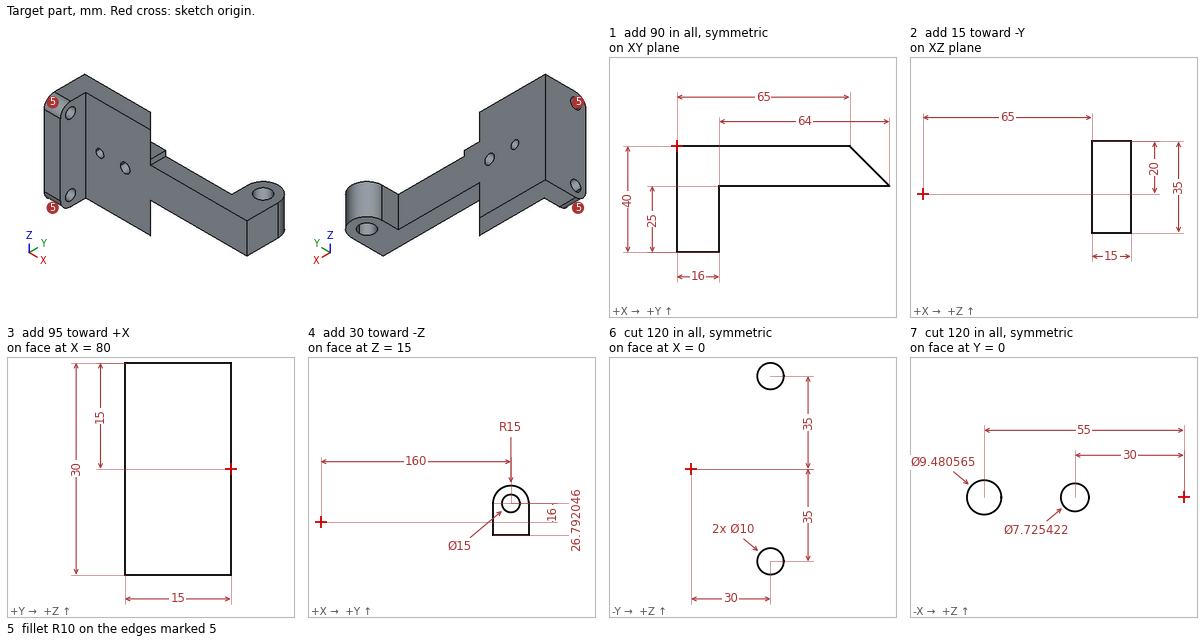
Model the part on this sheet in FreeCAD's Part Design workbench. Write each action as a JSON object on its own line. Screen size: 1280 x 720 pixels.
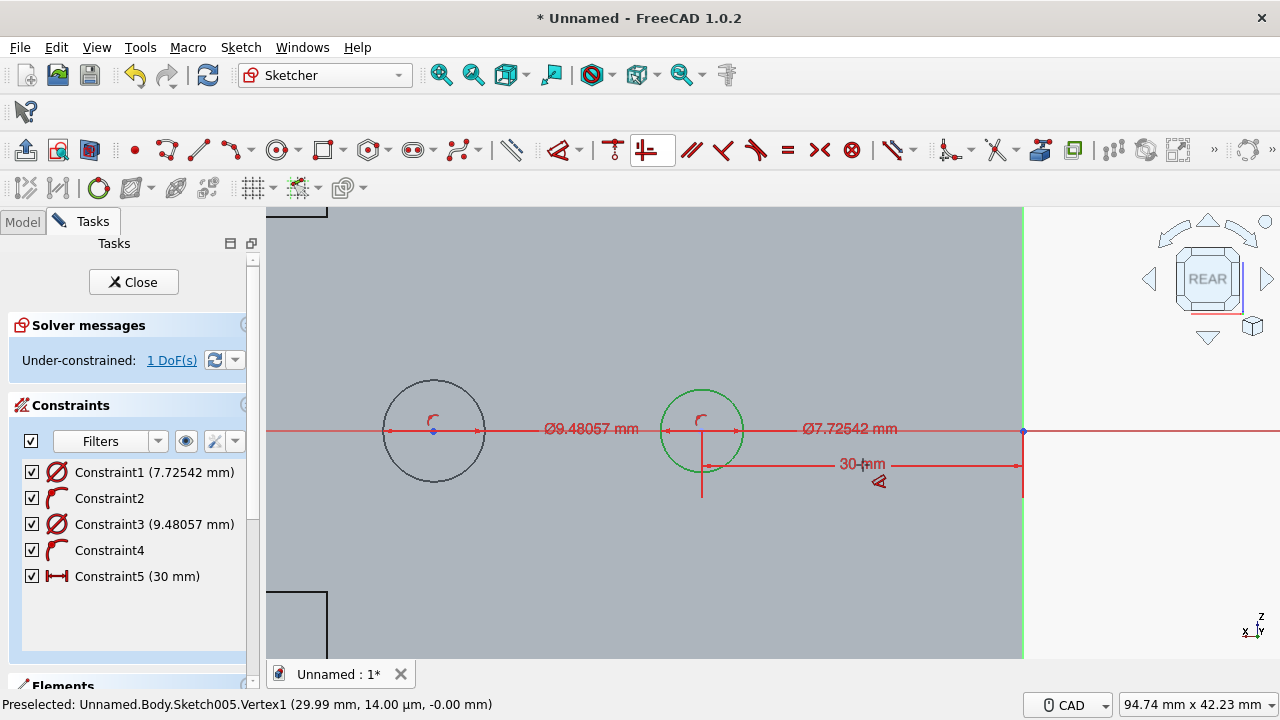
{"action": "left_click", "coordinate": [434, 431]}
{"action": "left_click", "coordinate": [593, 465]}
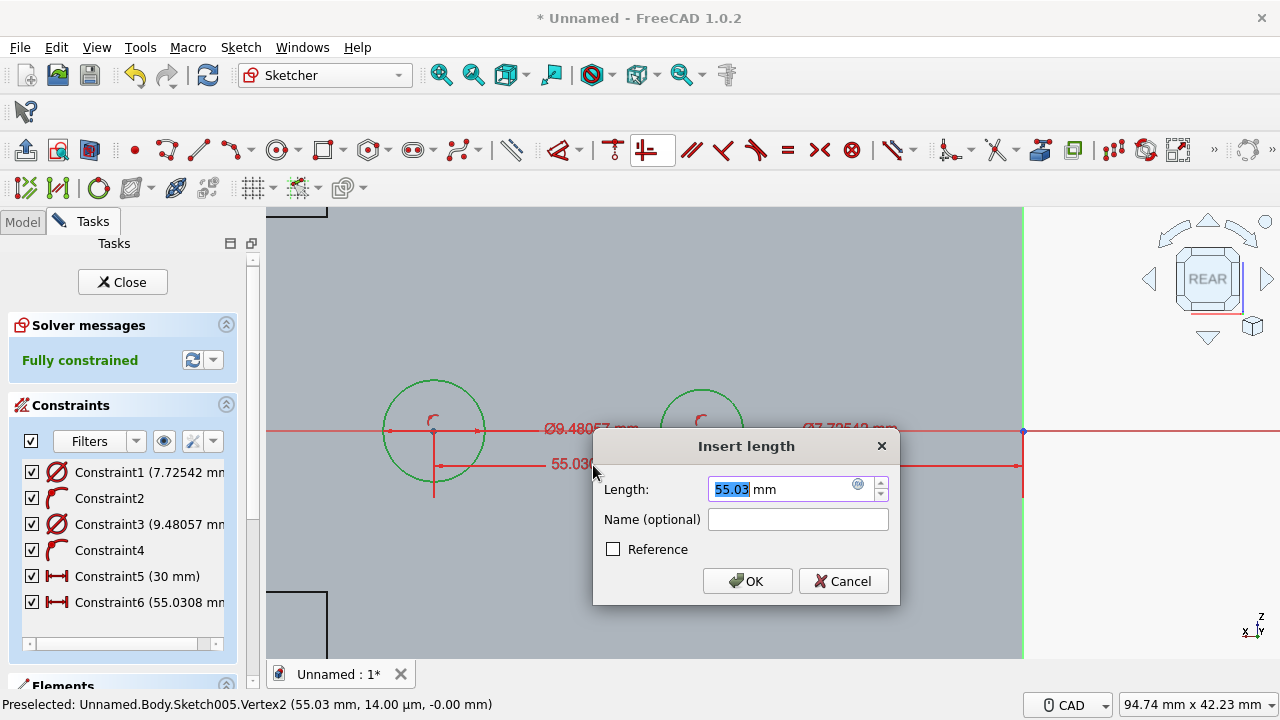
{"action": "type", "text": "55"}
{"action": "key", "text": "Return"}
{"action": "key", "text": "Escape"}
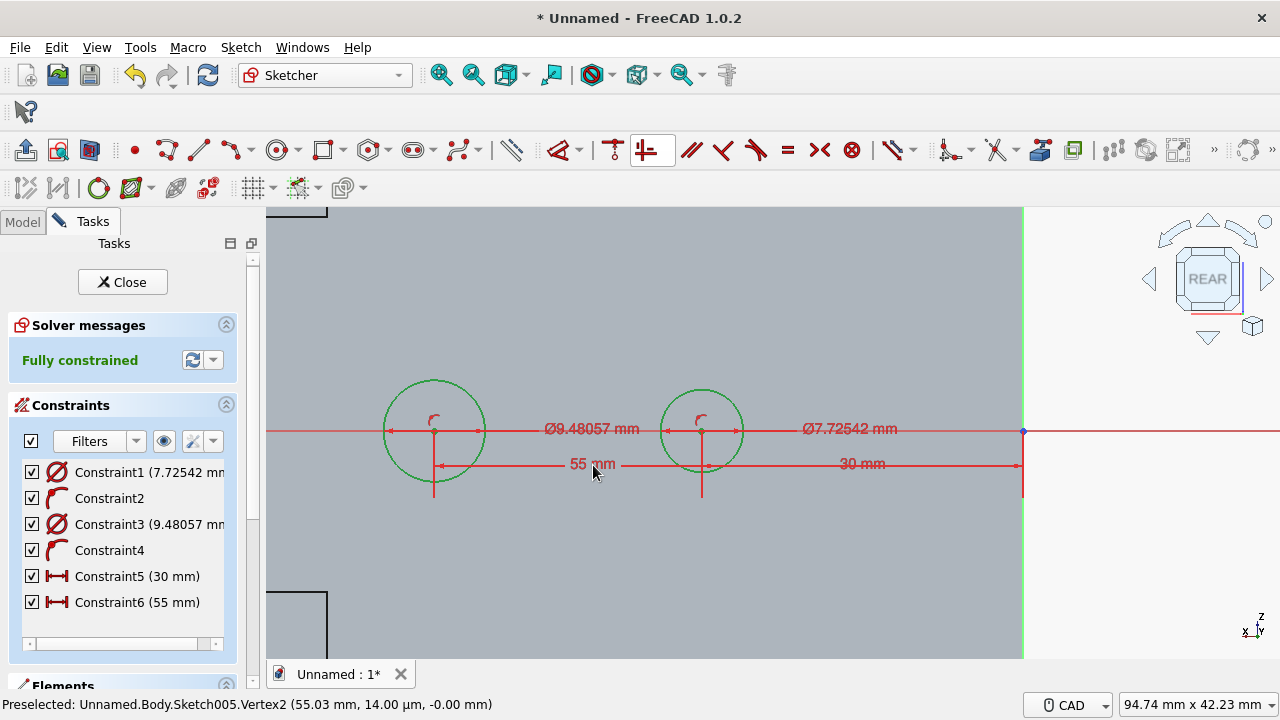
{"action": "left_click", "coordinate": [123, 282]}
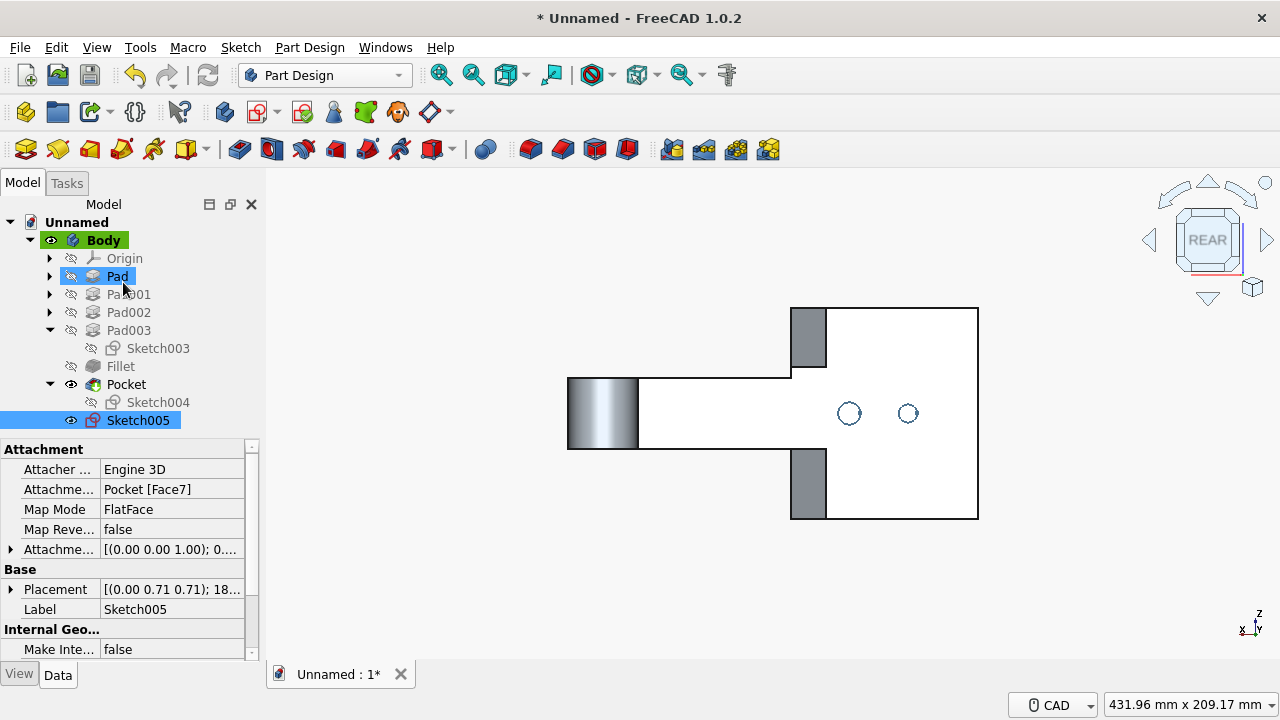
{"action": "left_click", "coordinate": [240, 150]}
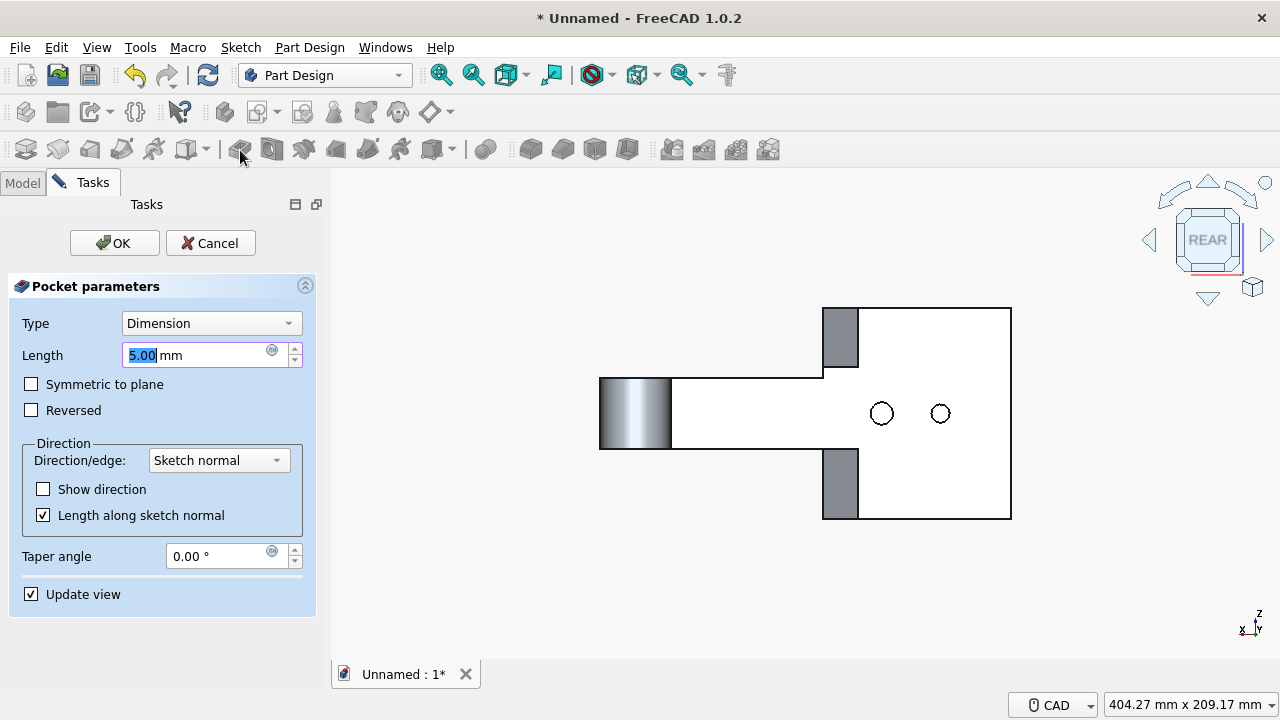
{"action": "type", "text": "120"}
{"action": "key", "text": "Tab"}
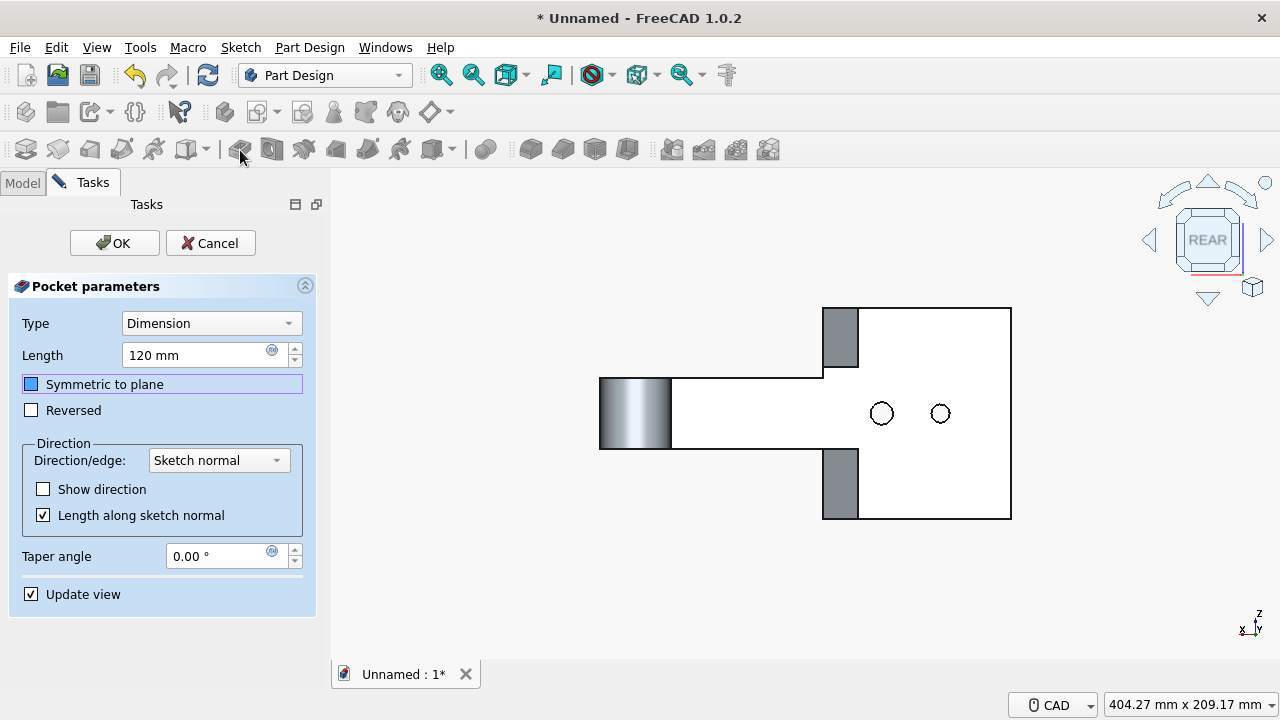
{"action": "left_click", "coordinate": [30, 384]}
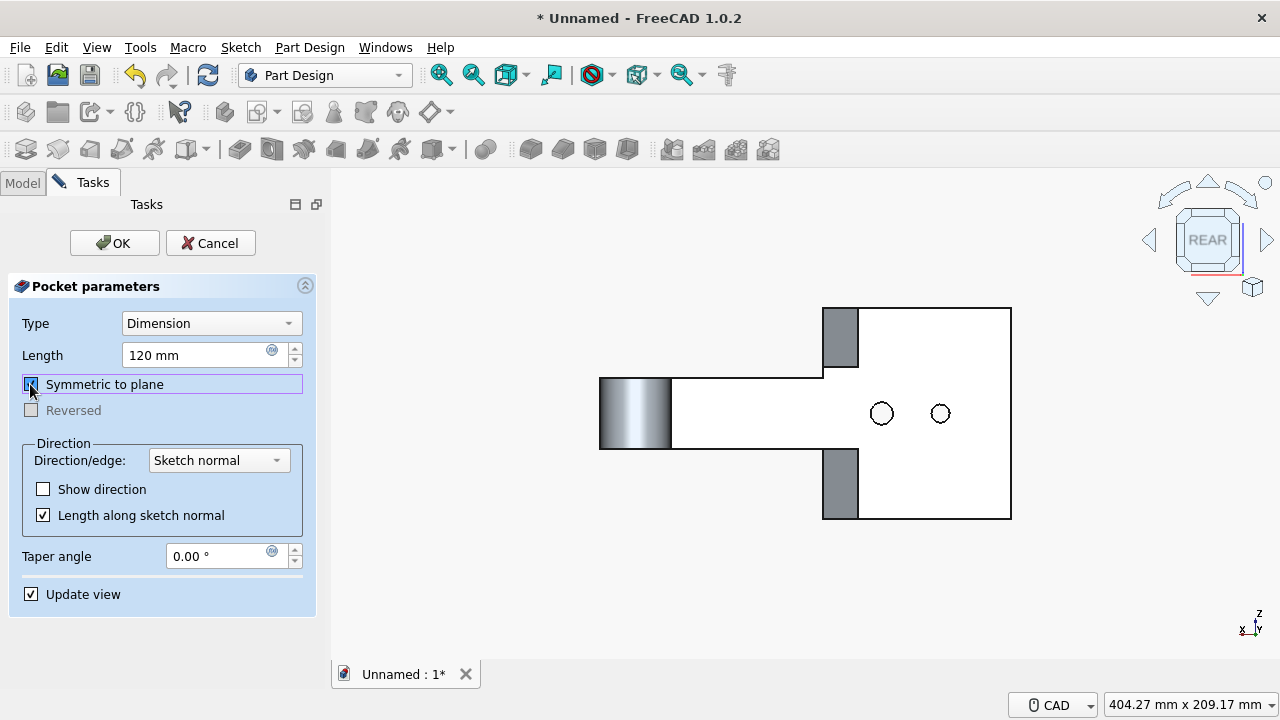
{"action": "left_click", "coordinate": [115, 243]}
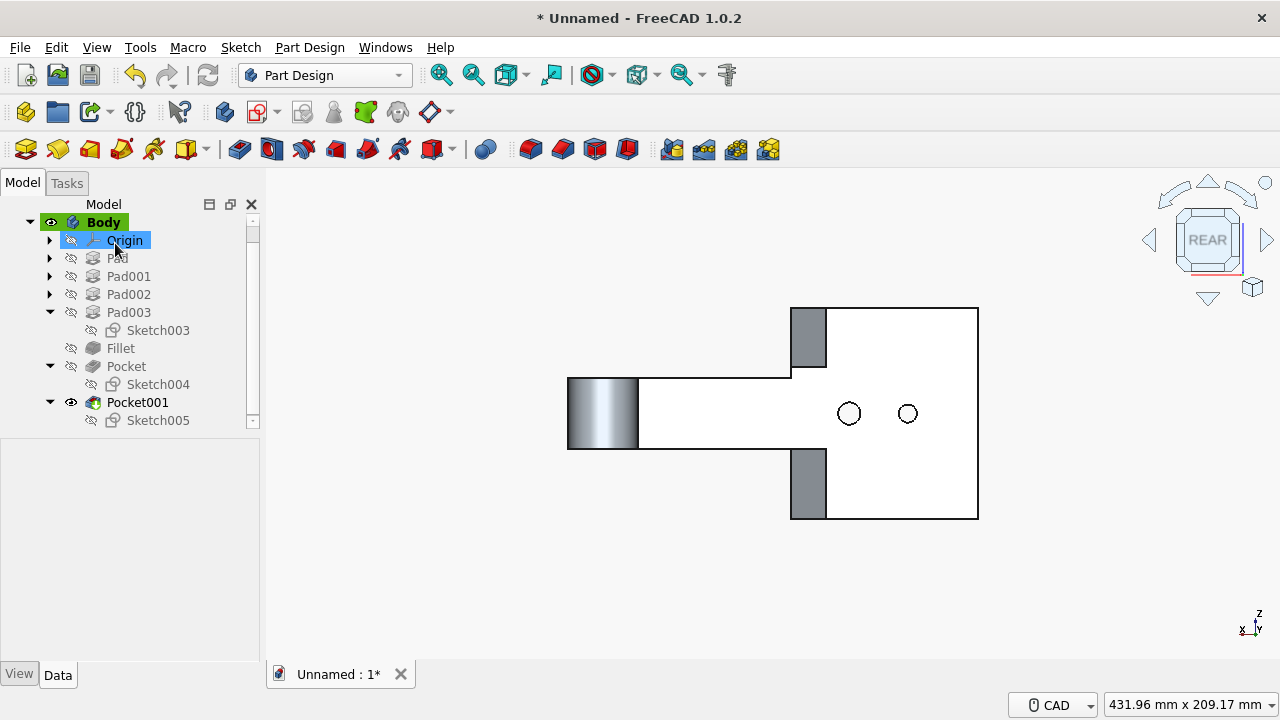
{"action": "key", "text": "0"}